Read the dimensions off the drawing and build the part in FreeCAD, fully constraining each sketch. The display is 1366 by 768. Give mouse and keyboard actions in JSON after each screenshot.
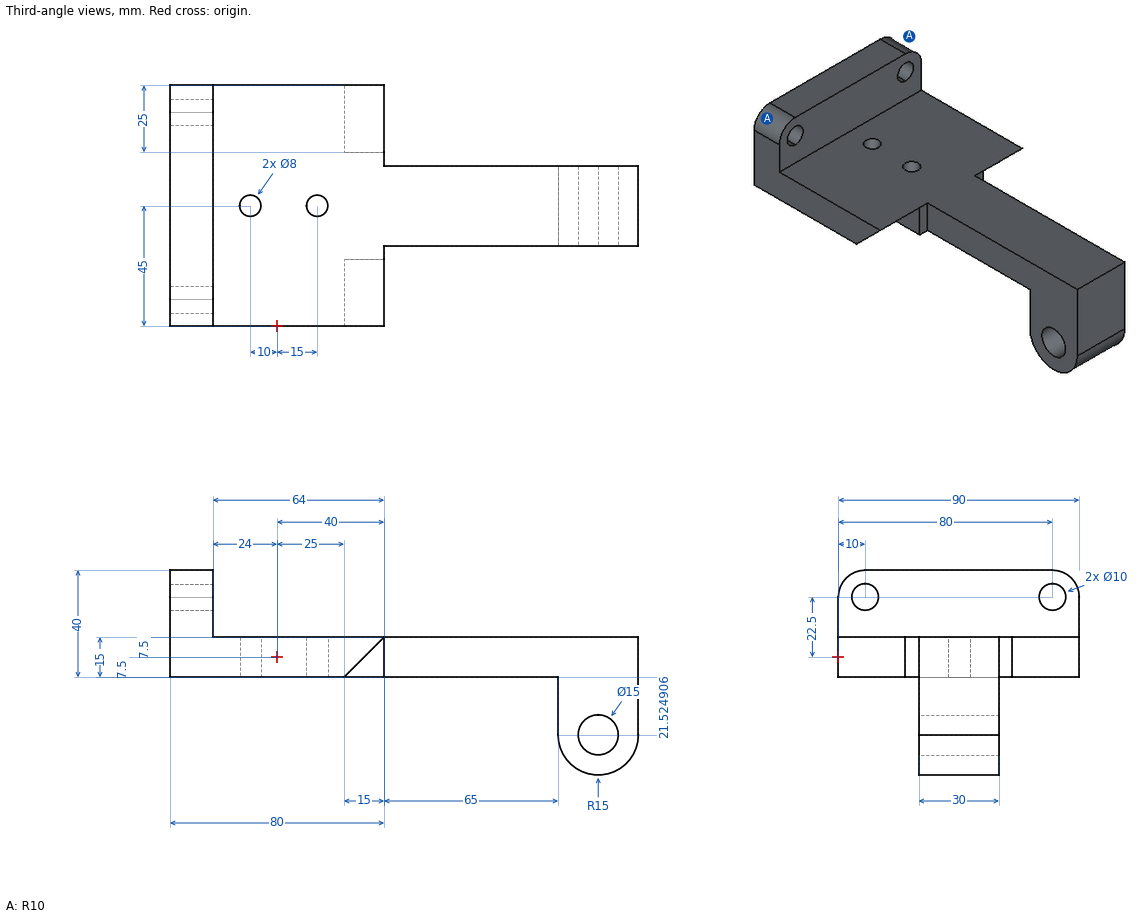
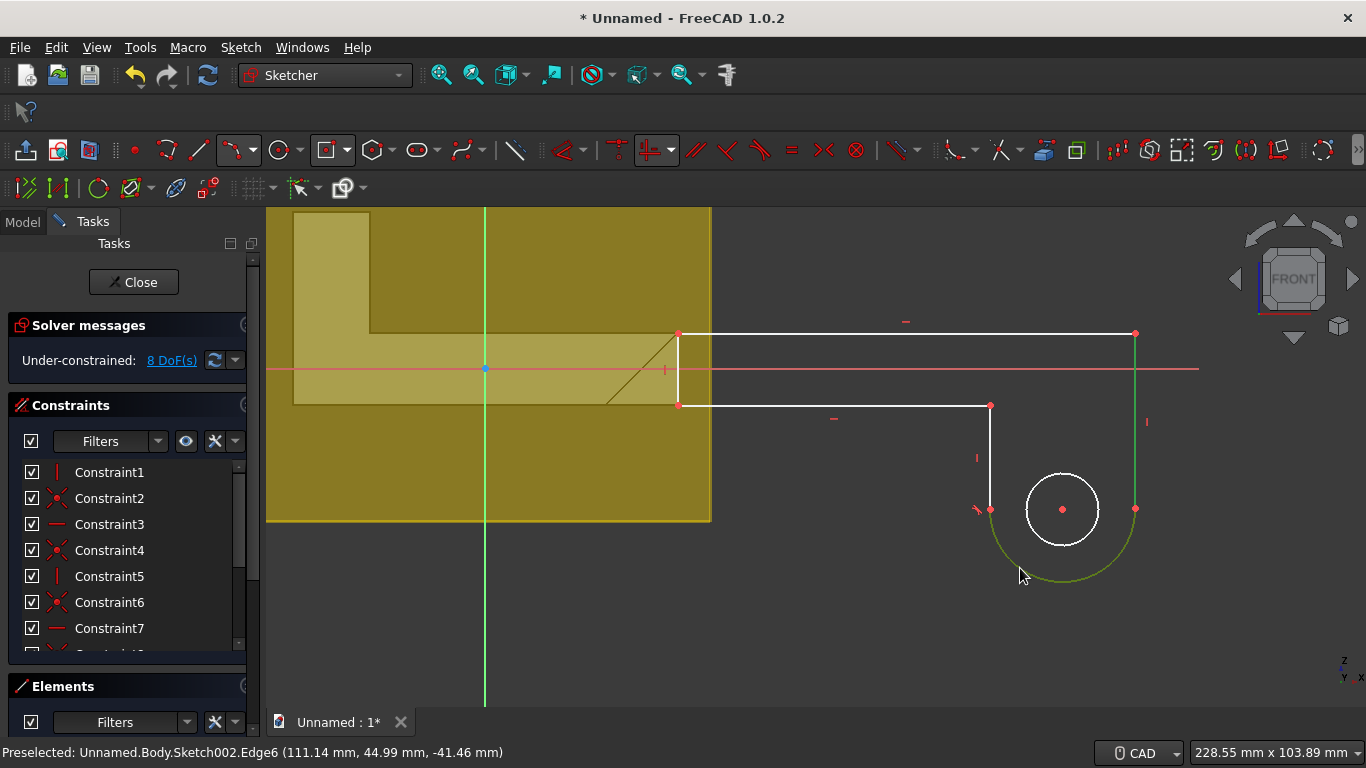
{"action": "left_click", "coordinate": [760, 150]}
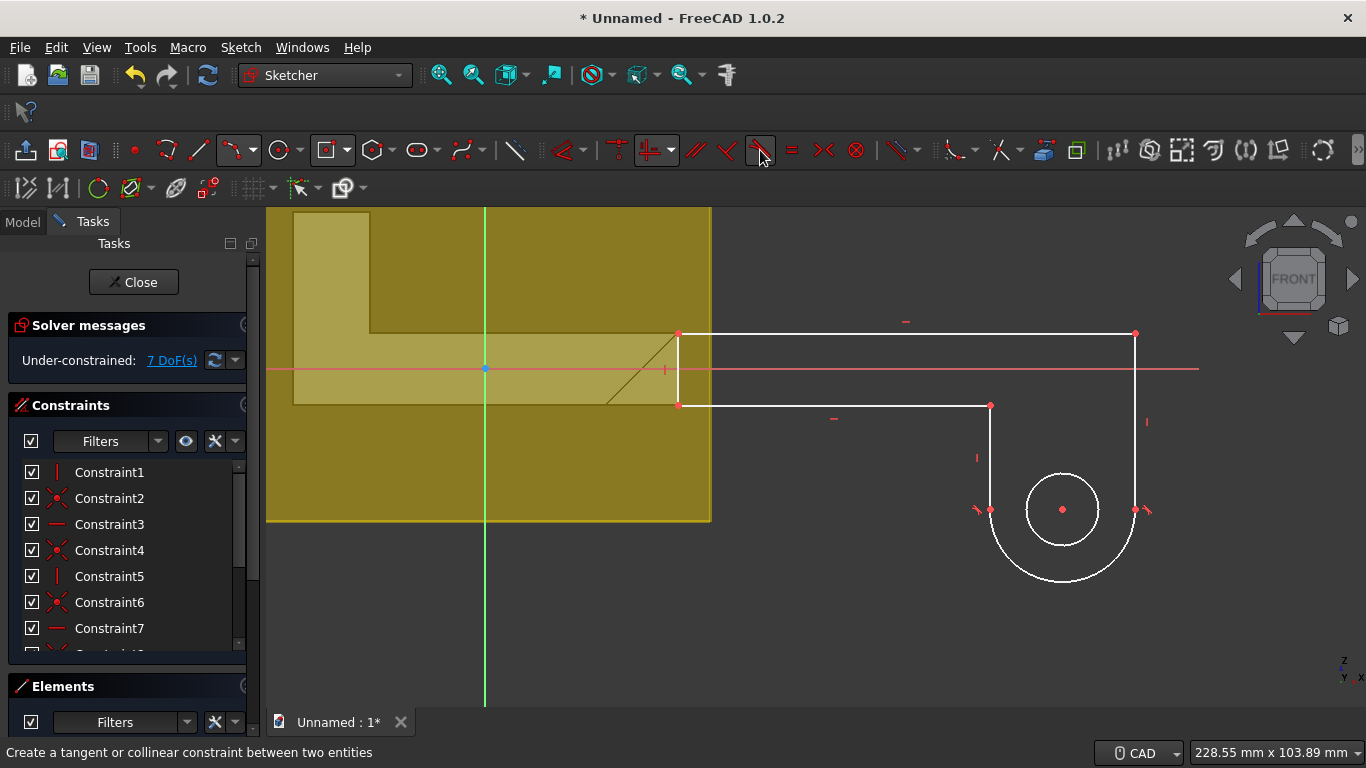
{"action": "left_click", "coordinate": [562, 150]}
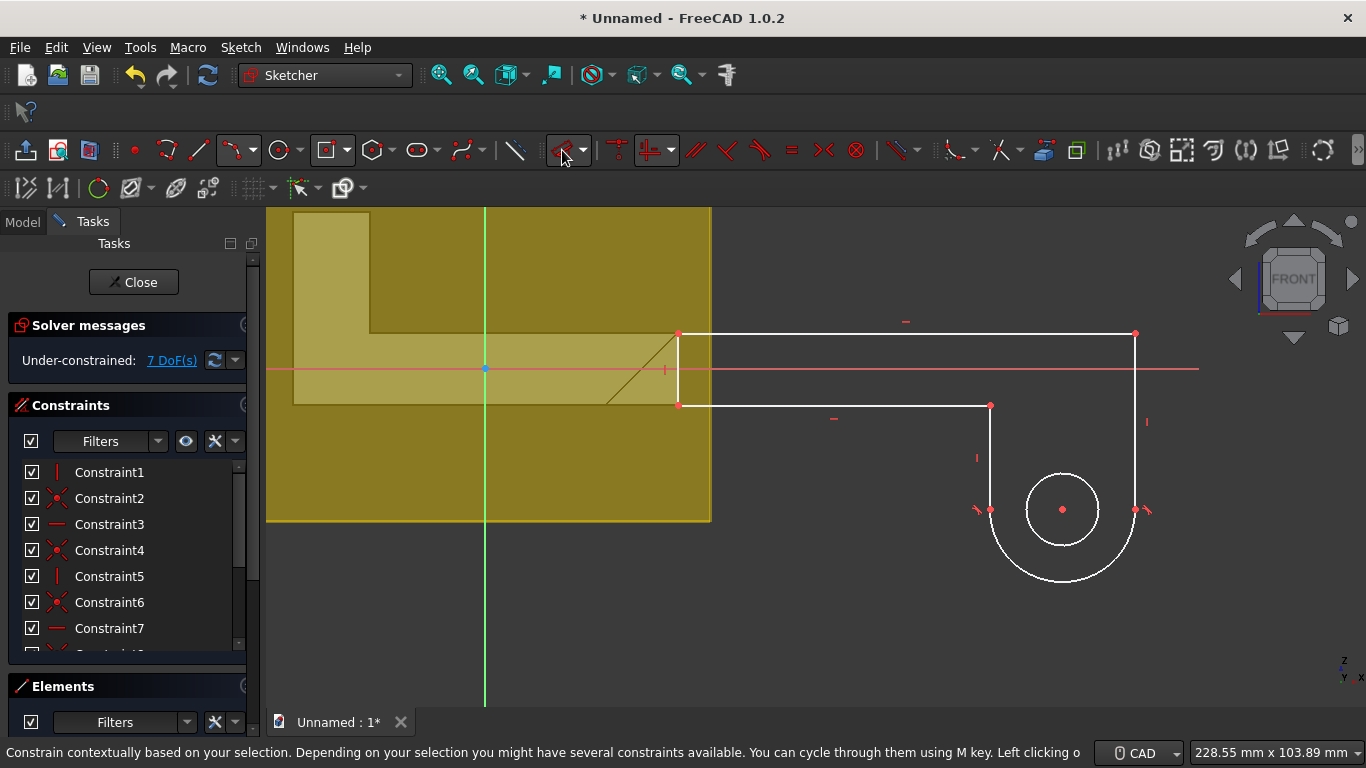
{"action": "left_click", "coordinate": [1020, 568]}
{"action": "left_click", "coordinate": [1001, 594]}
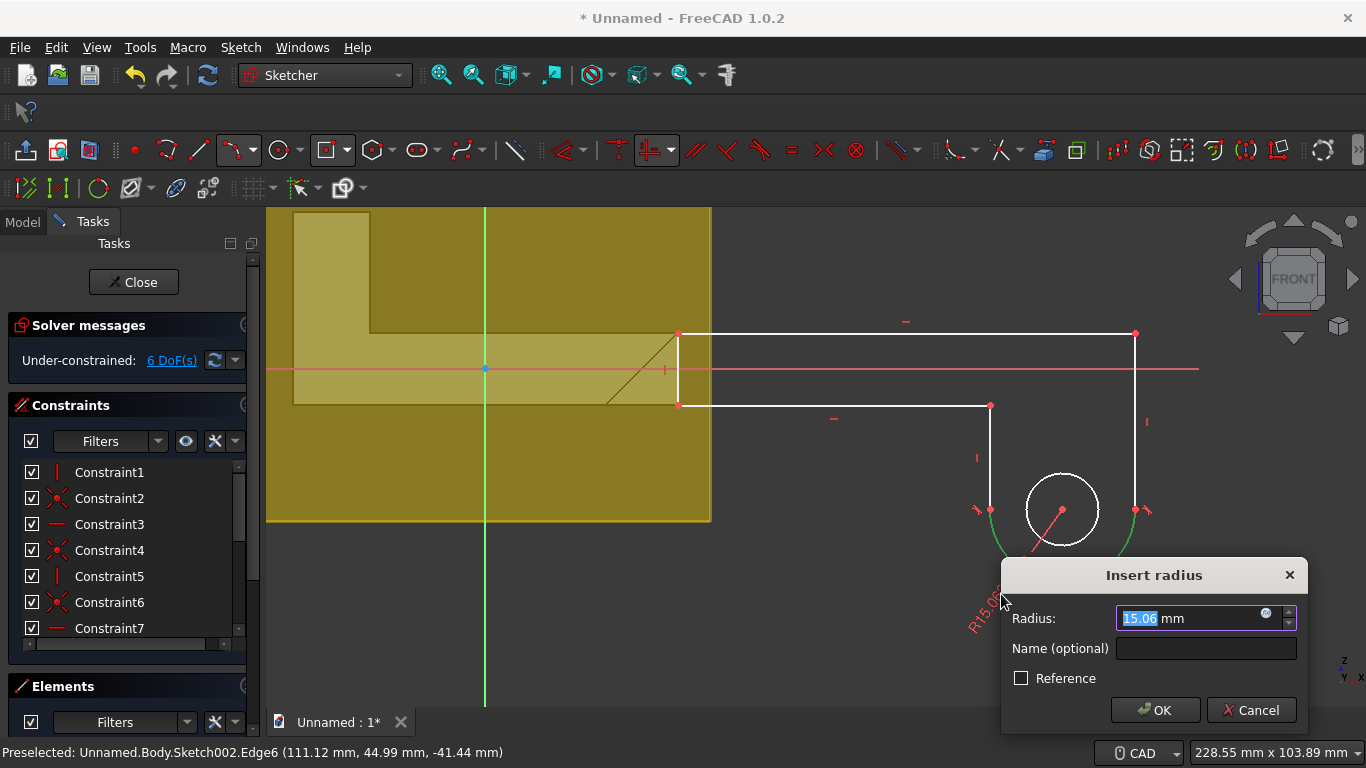
{"action": "type", "text": "15"}
{"action": "key", "text": "Return"}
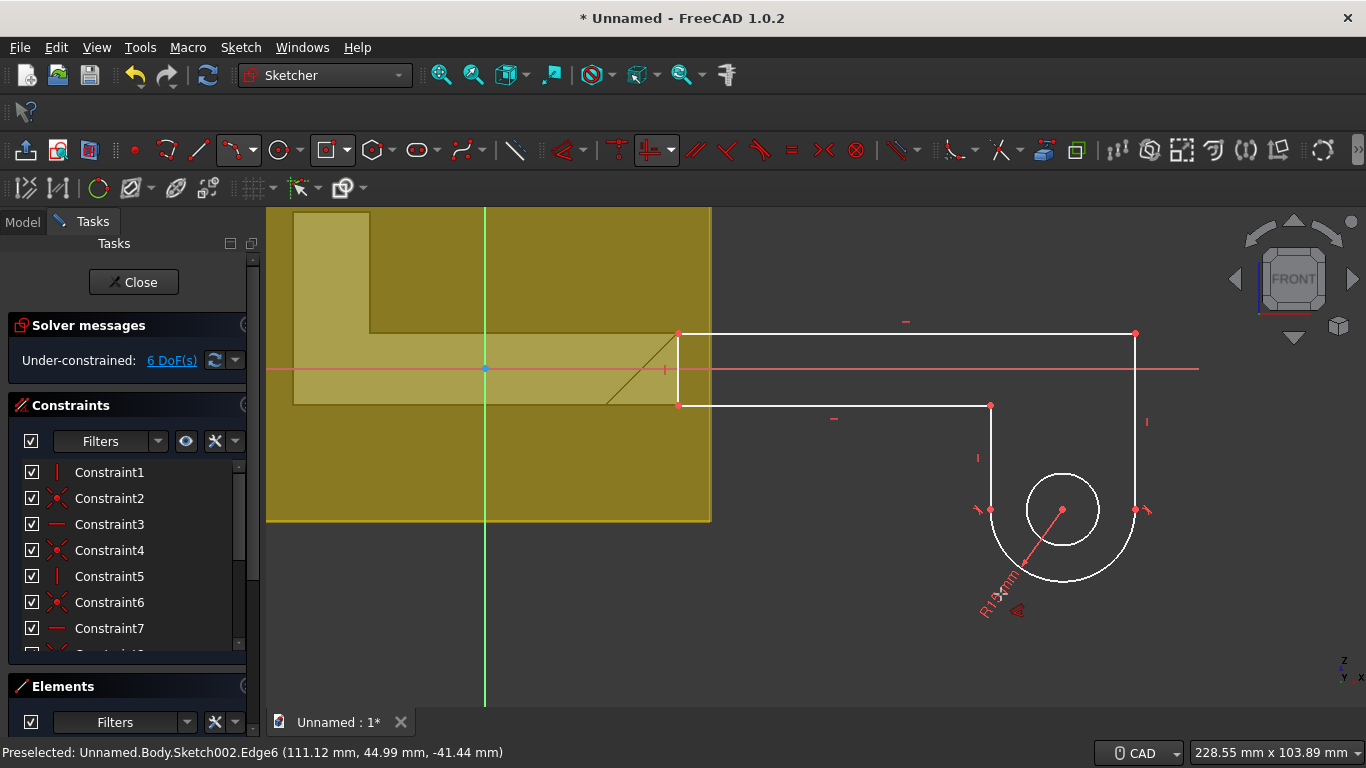
{"action": "left_click", "coordinate": [1088, 484]}
{"action": "left_click", "coordinate": [1110, 461]}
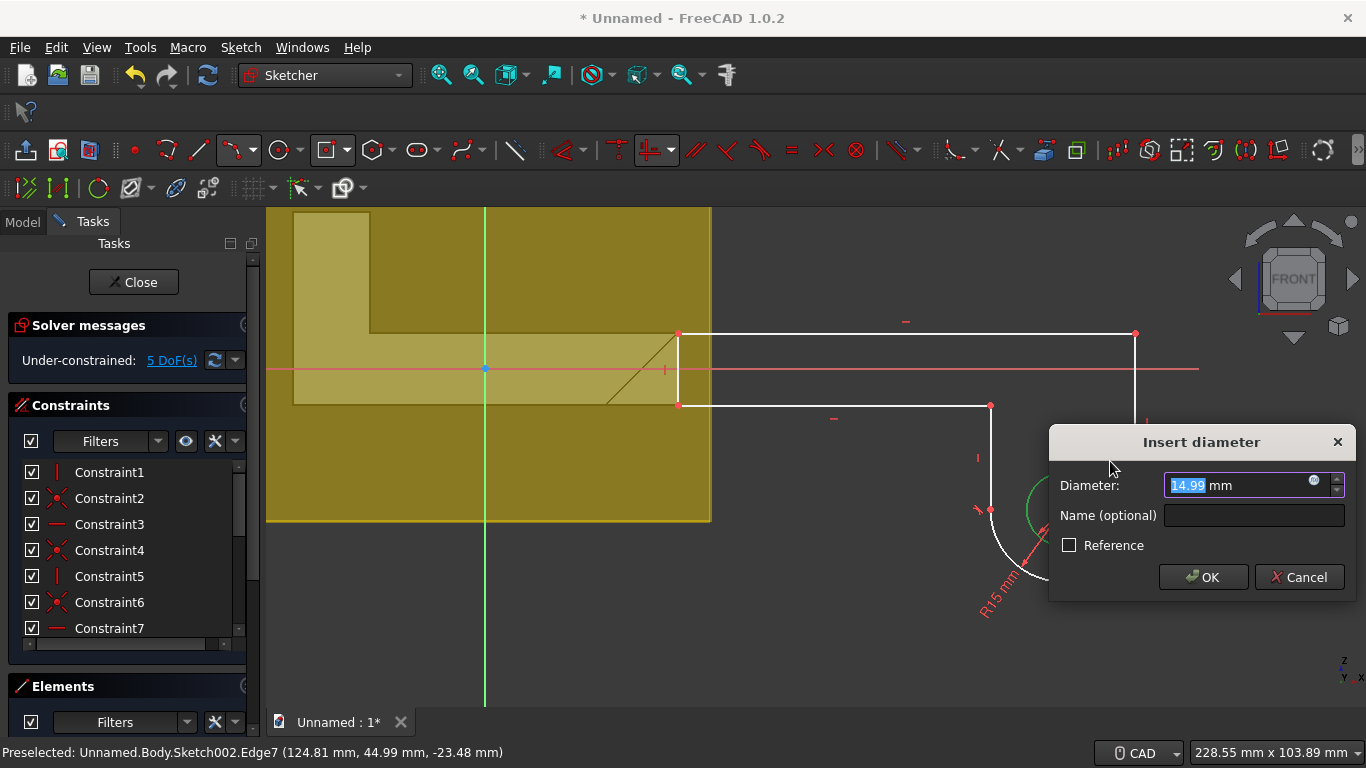
{"action": "type", "text": "15"}
{"action": "key", "text": "Return"}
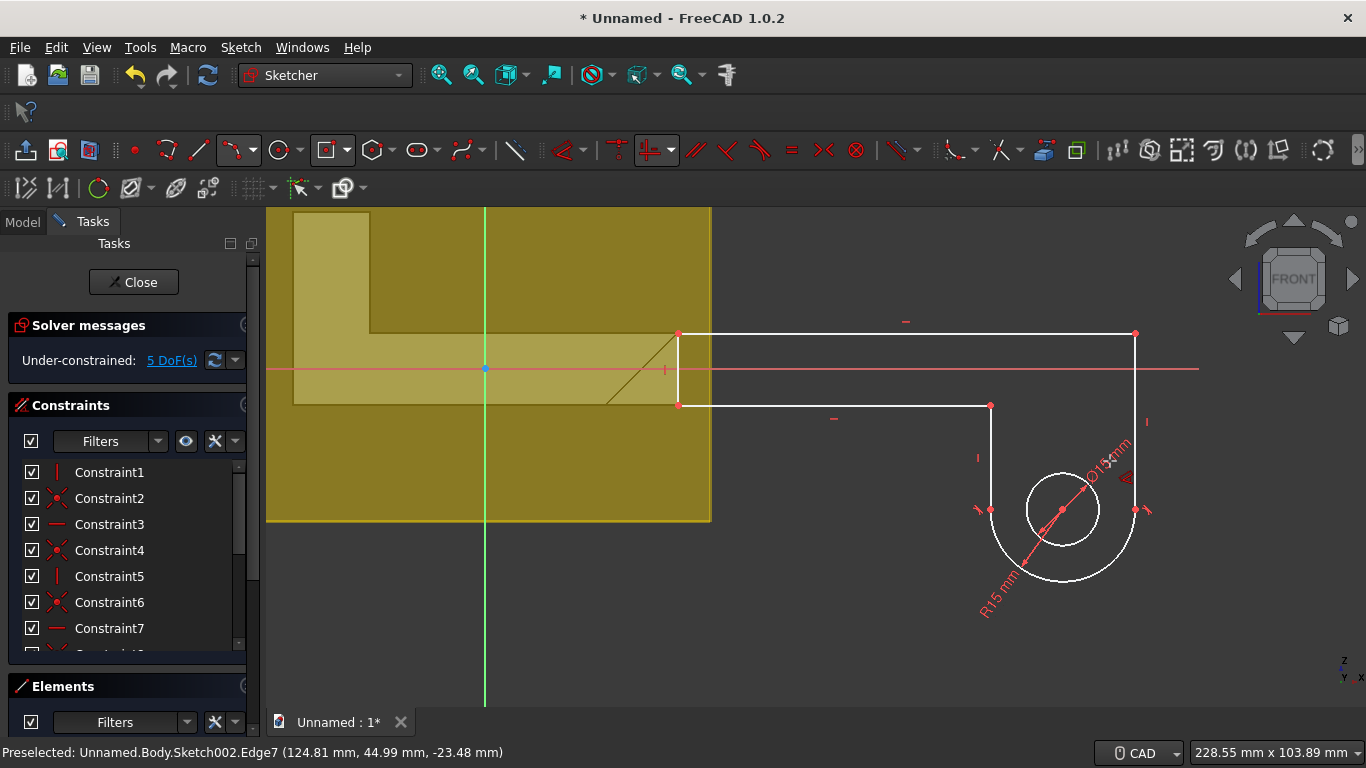
{"action": "left_click", "coordinate": [897, 406]}
{"action": "left_click", "coordinate": [834, 440]}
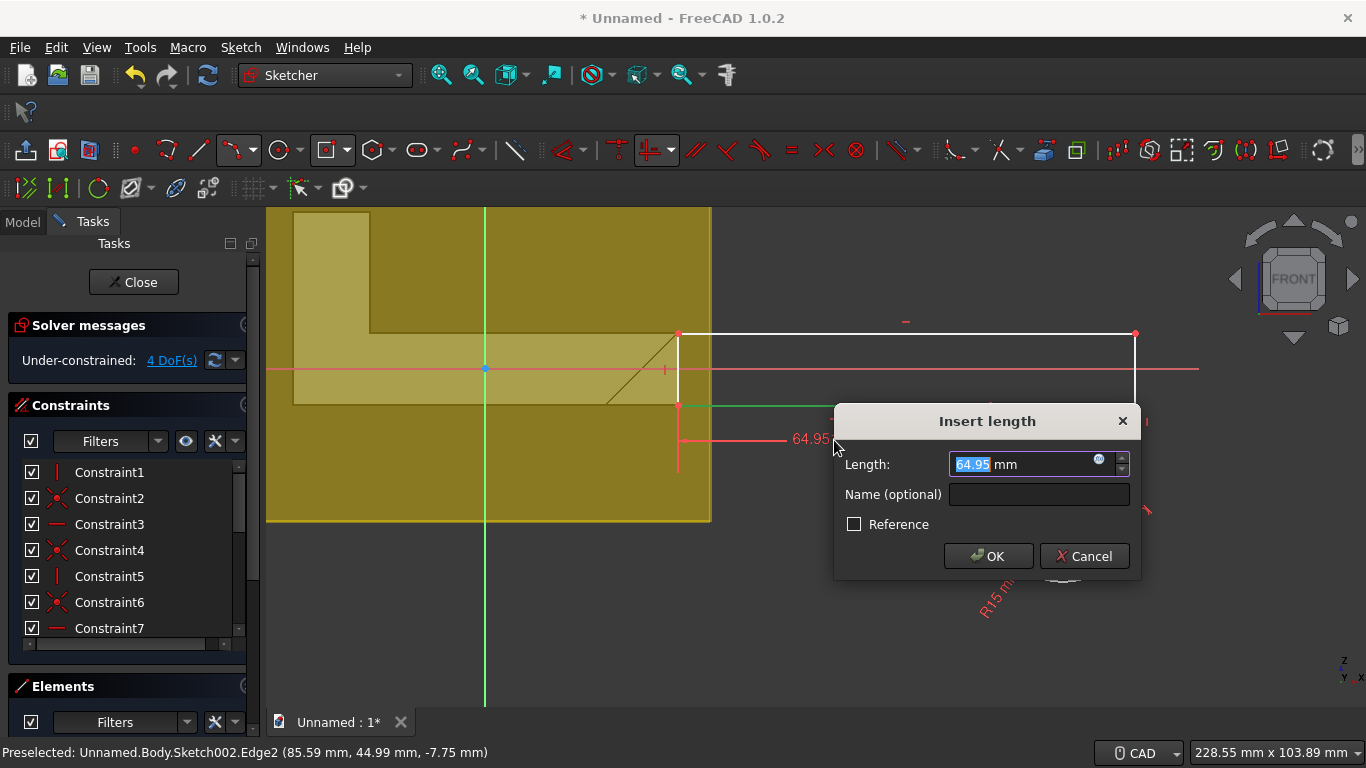
{"action": "type", "text": "65"}
{"action": "key", "text": "Return"}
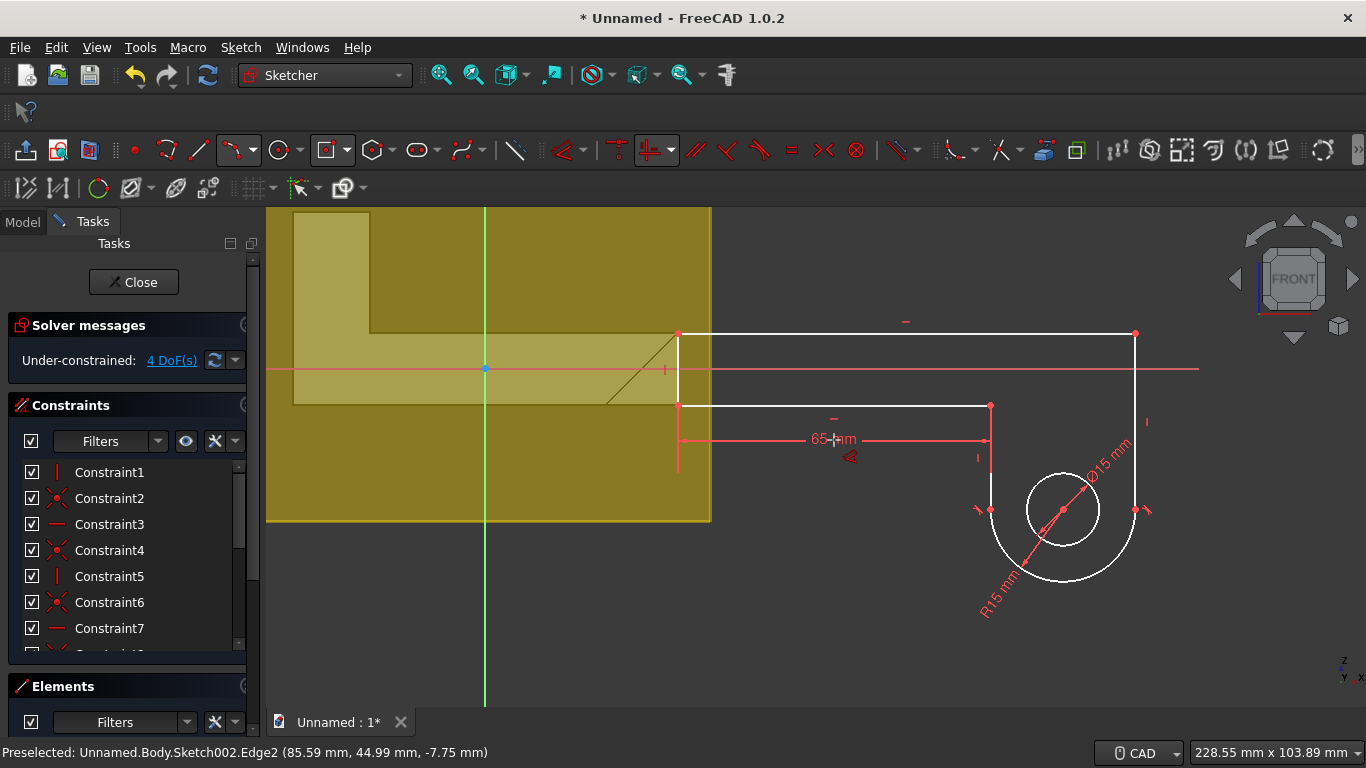
{"action": "left_click", "coordinate": [678, 384]}
{"action": "left_click", "coordinate": [644, 353]}